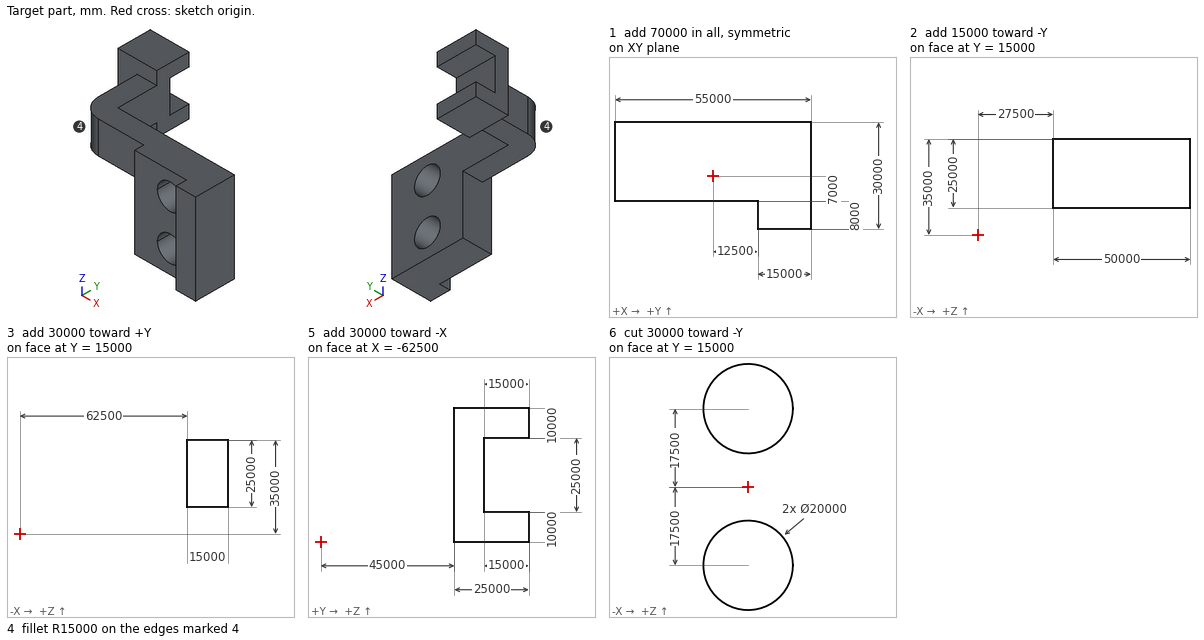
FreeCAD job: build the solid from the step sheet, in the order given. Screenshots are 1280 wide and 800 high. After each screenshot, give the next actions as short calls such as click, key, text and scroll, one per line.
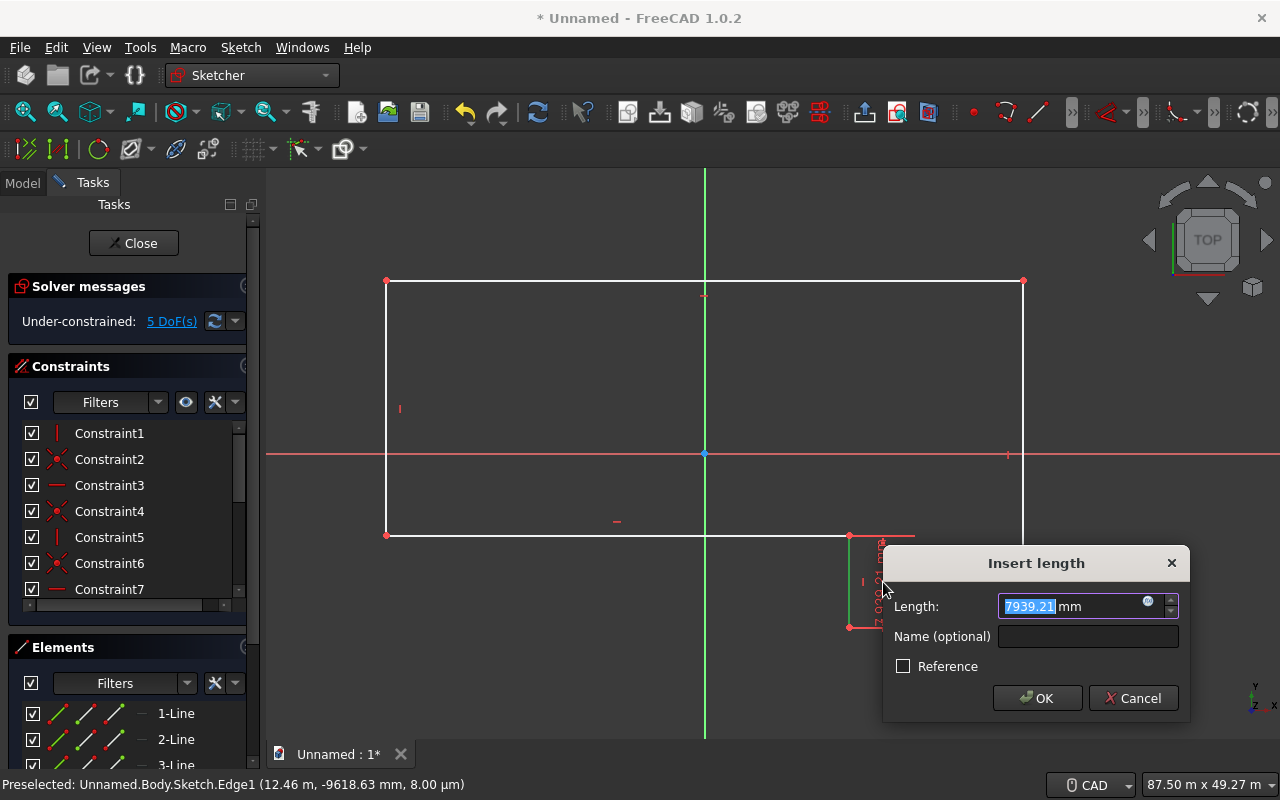
text(8000)
key(Return)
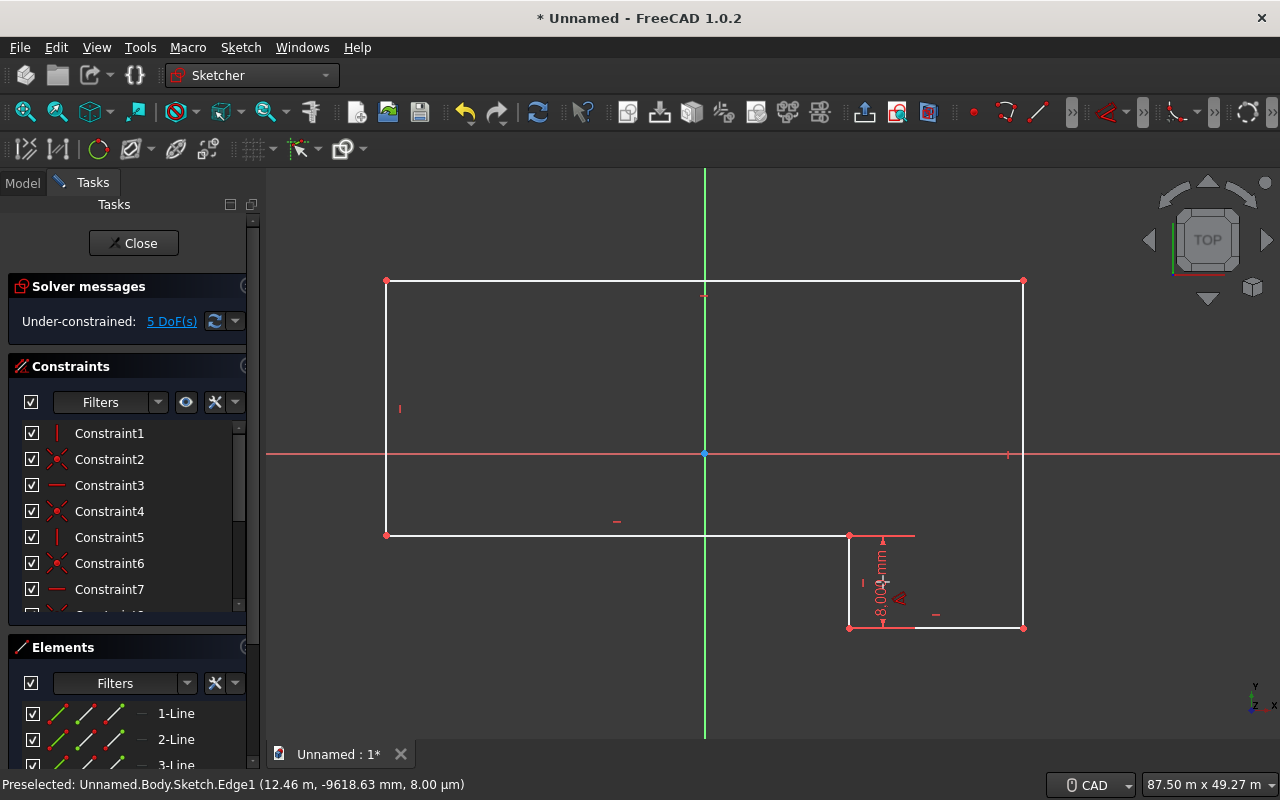
click(901, 628)
click(936, 662)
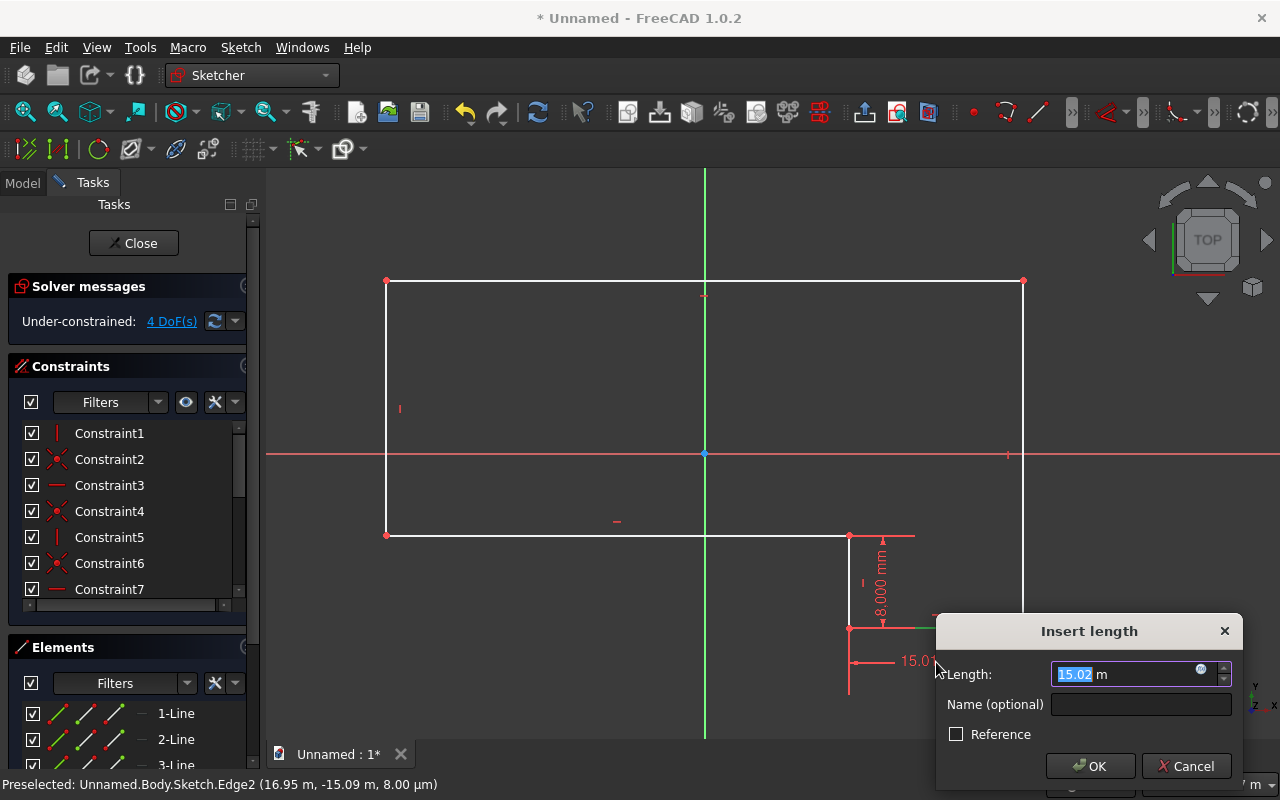
key(ctrl+a)
text(15000 mm)
key(Return)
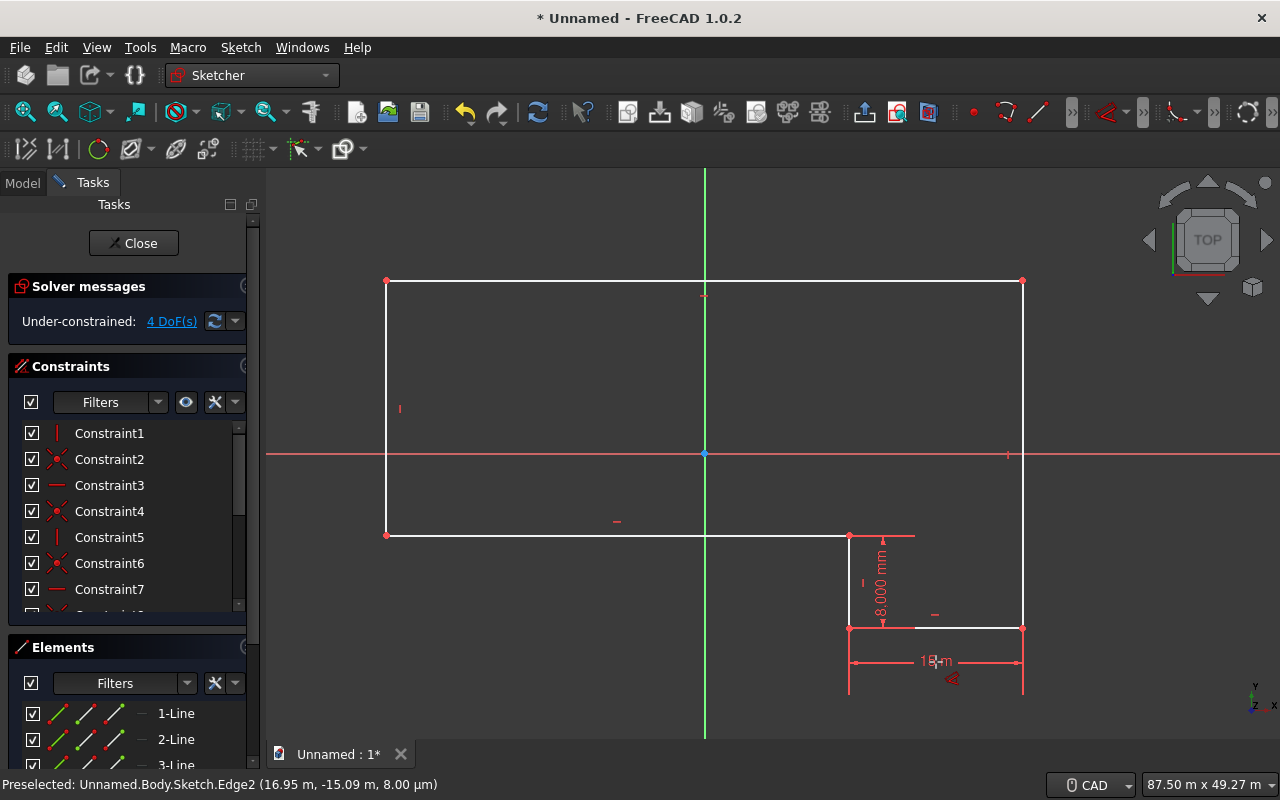
click(1023, 524)
click(1057, 375)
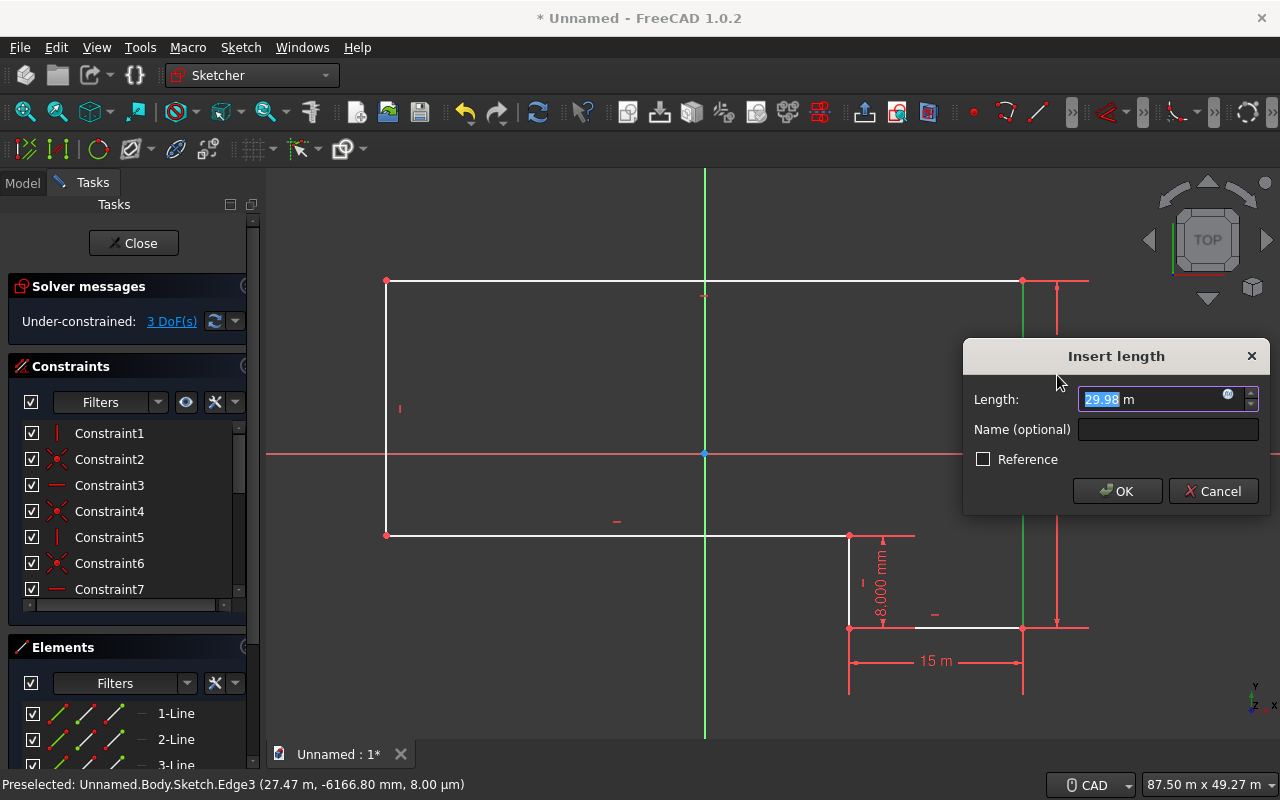
key(ctrl+a)
text(30000 mm)
key(Return)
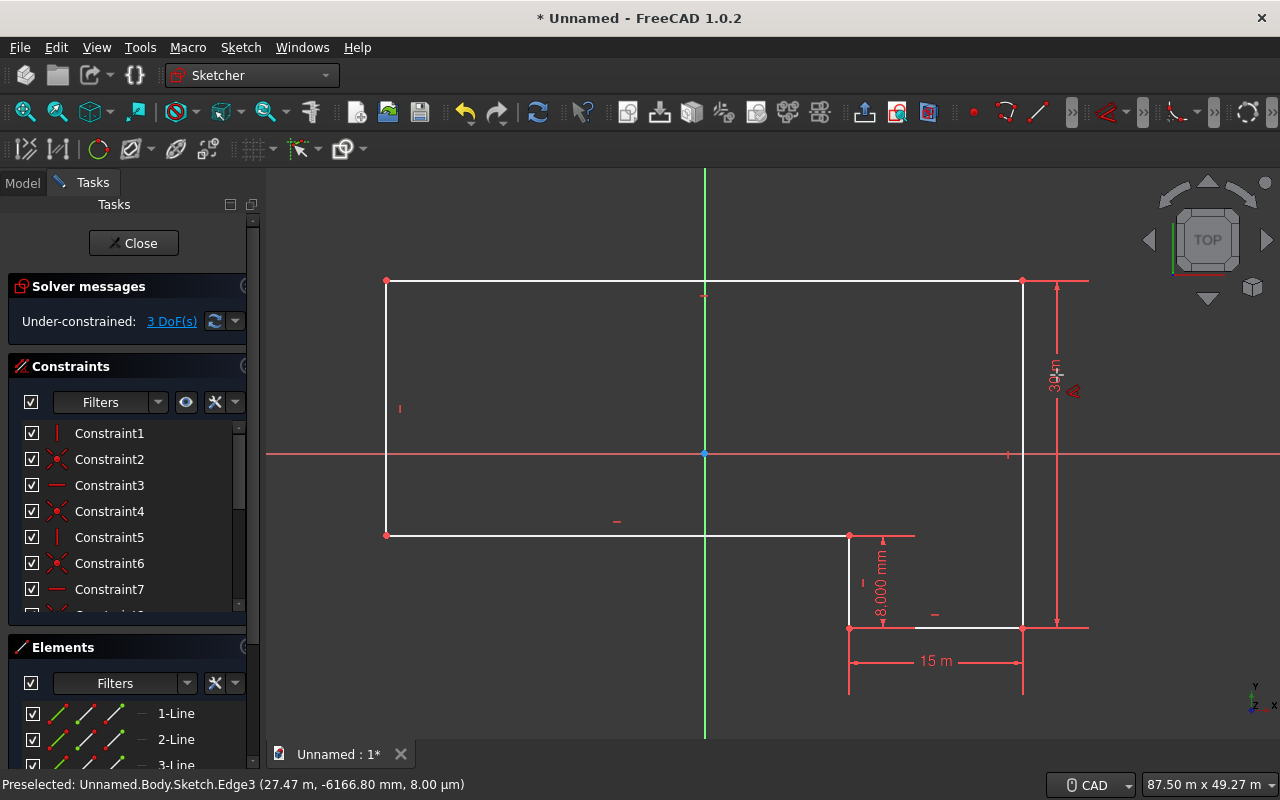
click(832, 281)
click(558, 247)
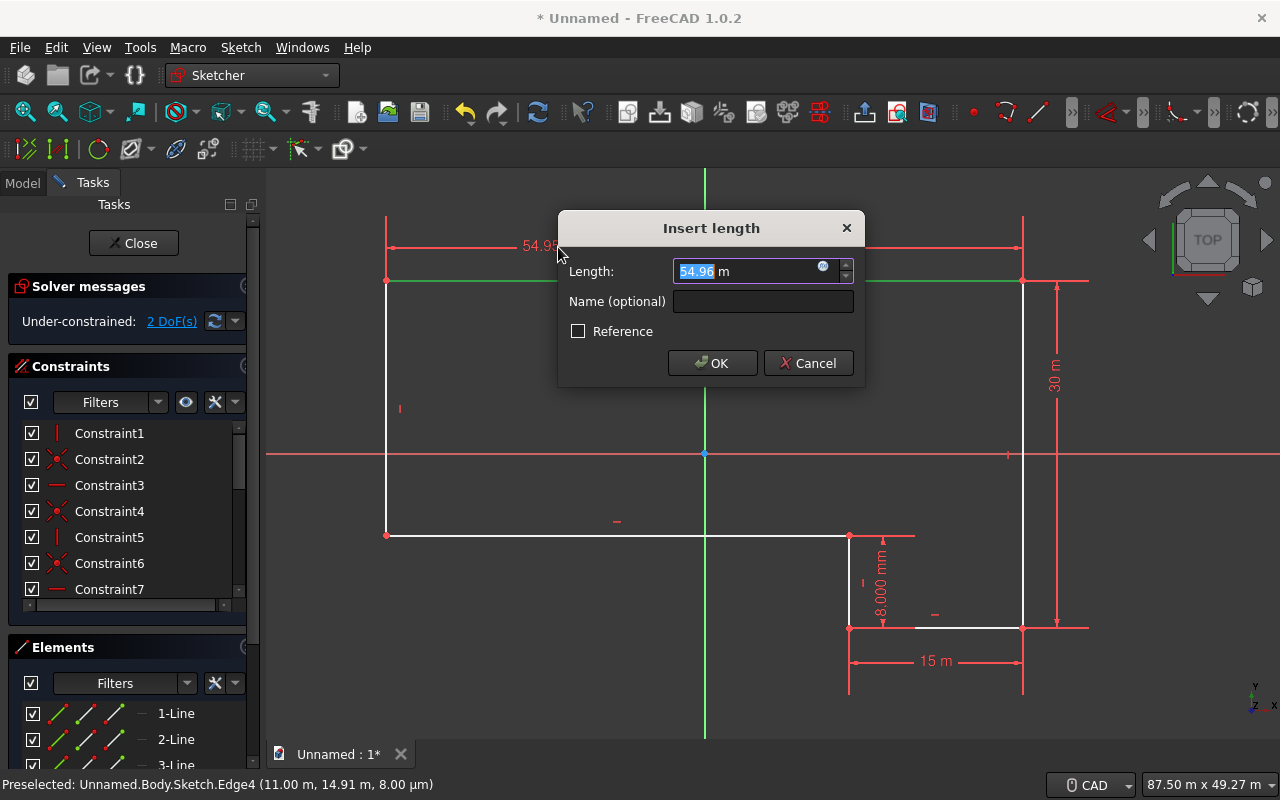
key(ctrl+a)
text(55000 mm)
key(Return)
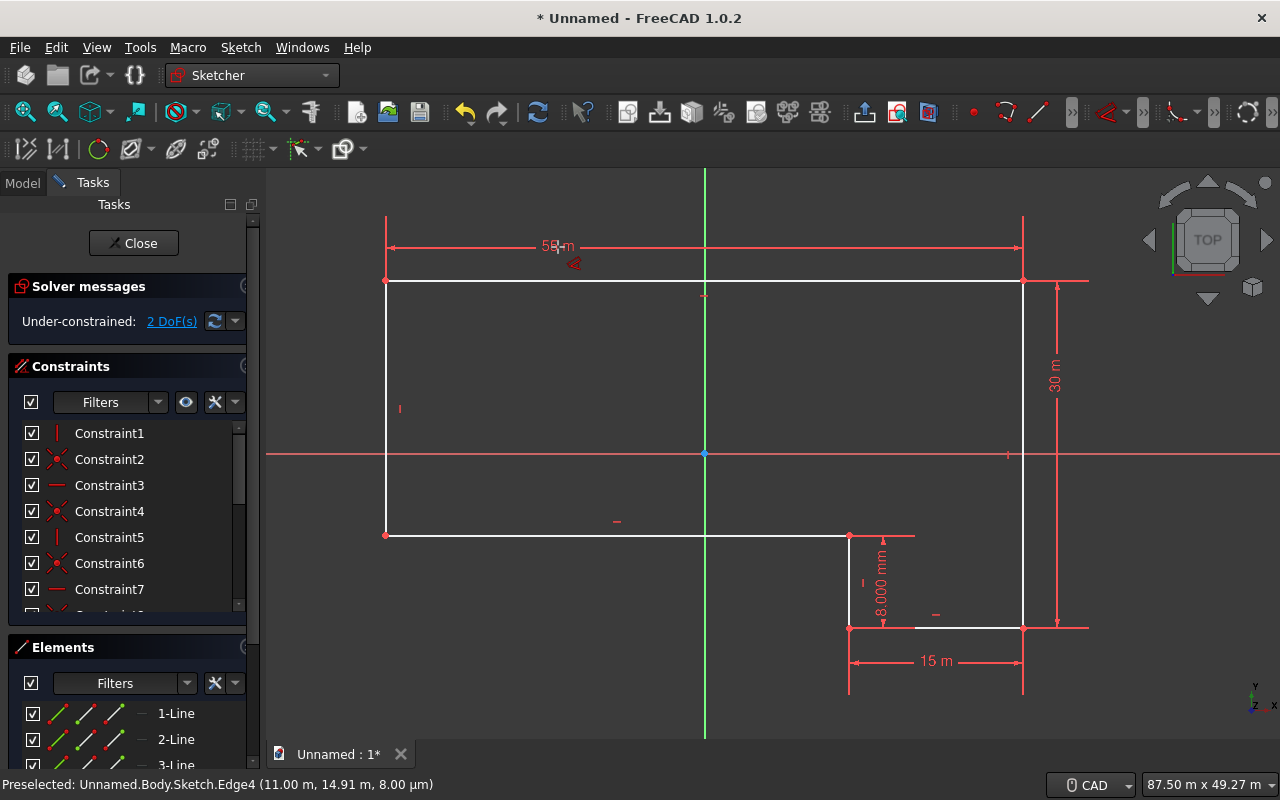
click(849, 536)
click(883, 495)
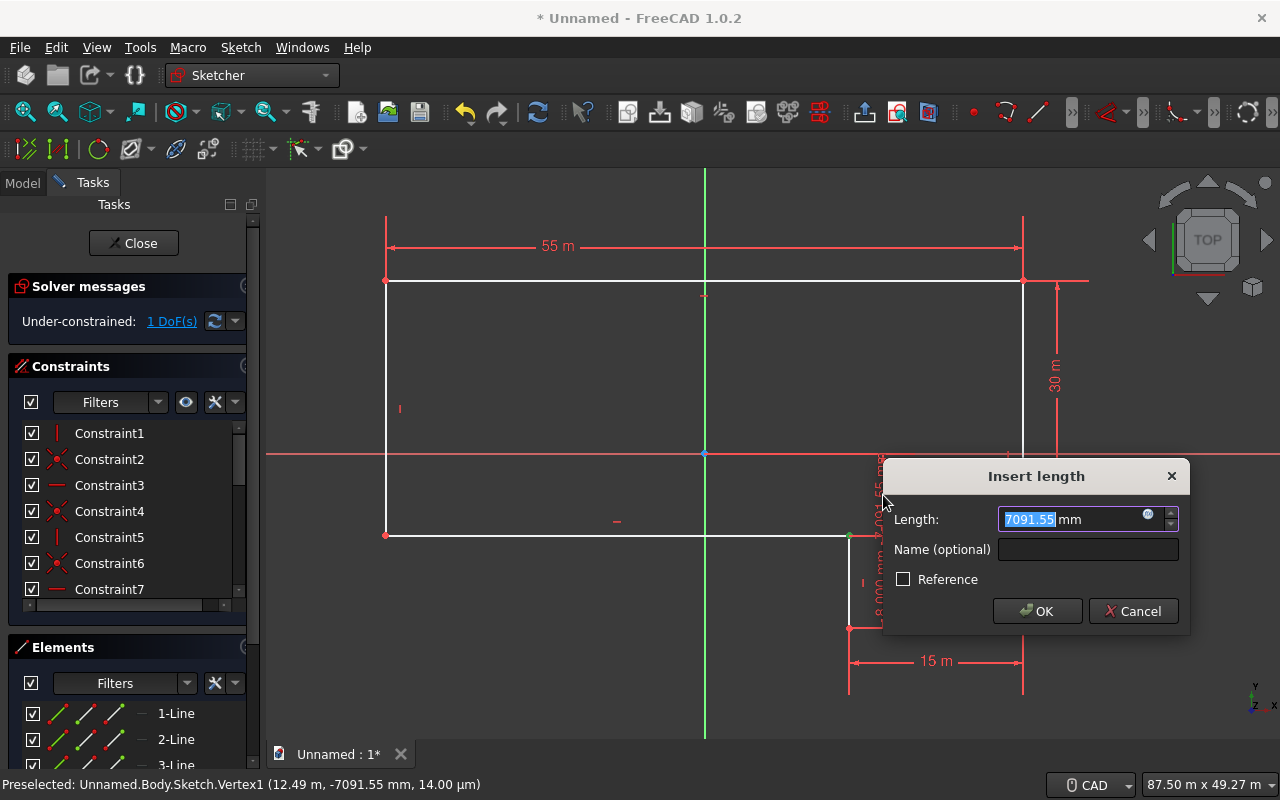
text(7000)
key(Return)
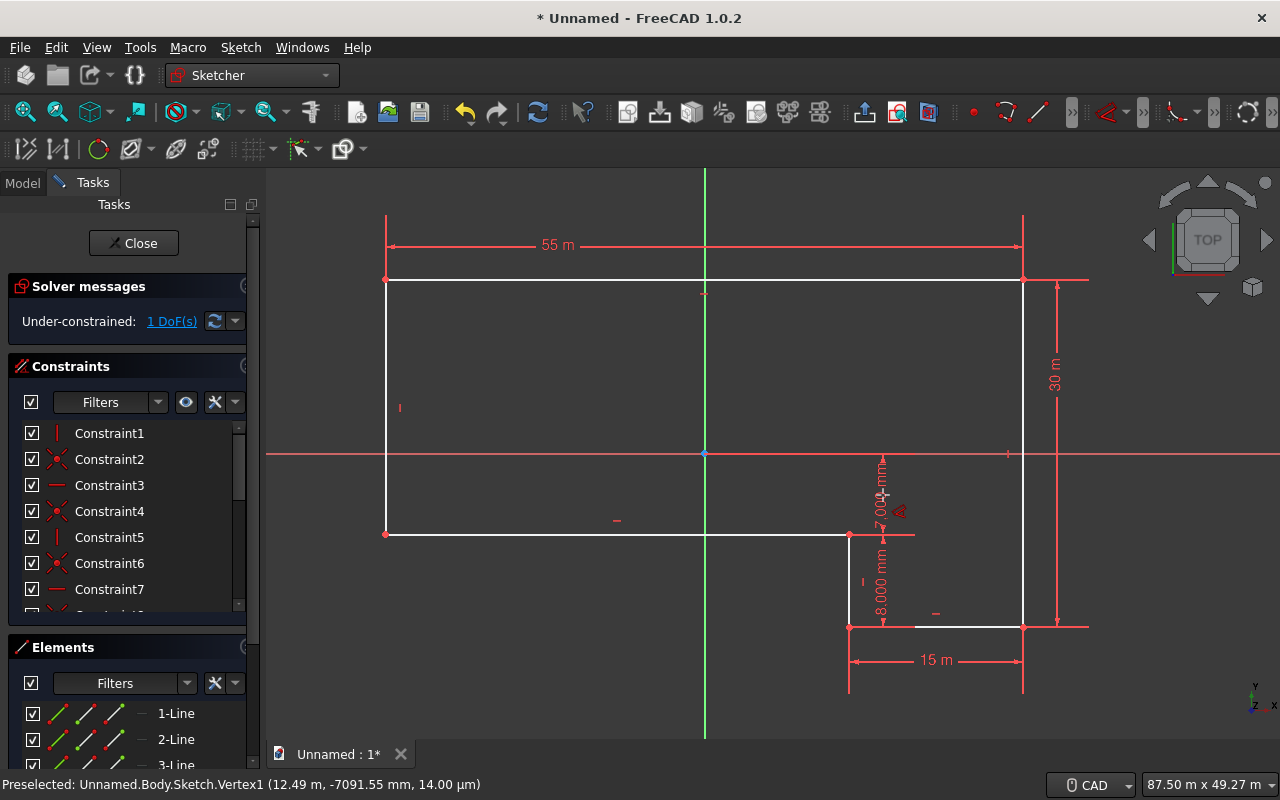
click(849, 535)
click(777, 569)